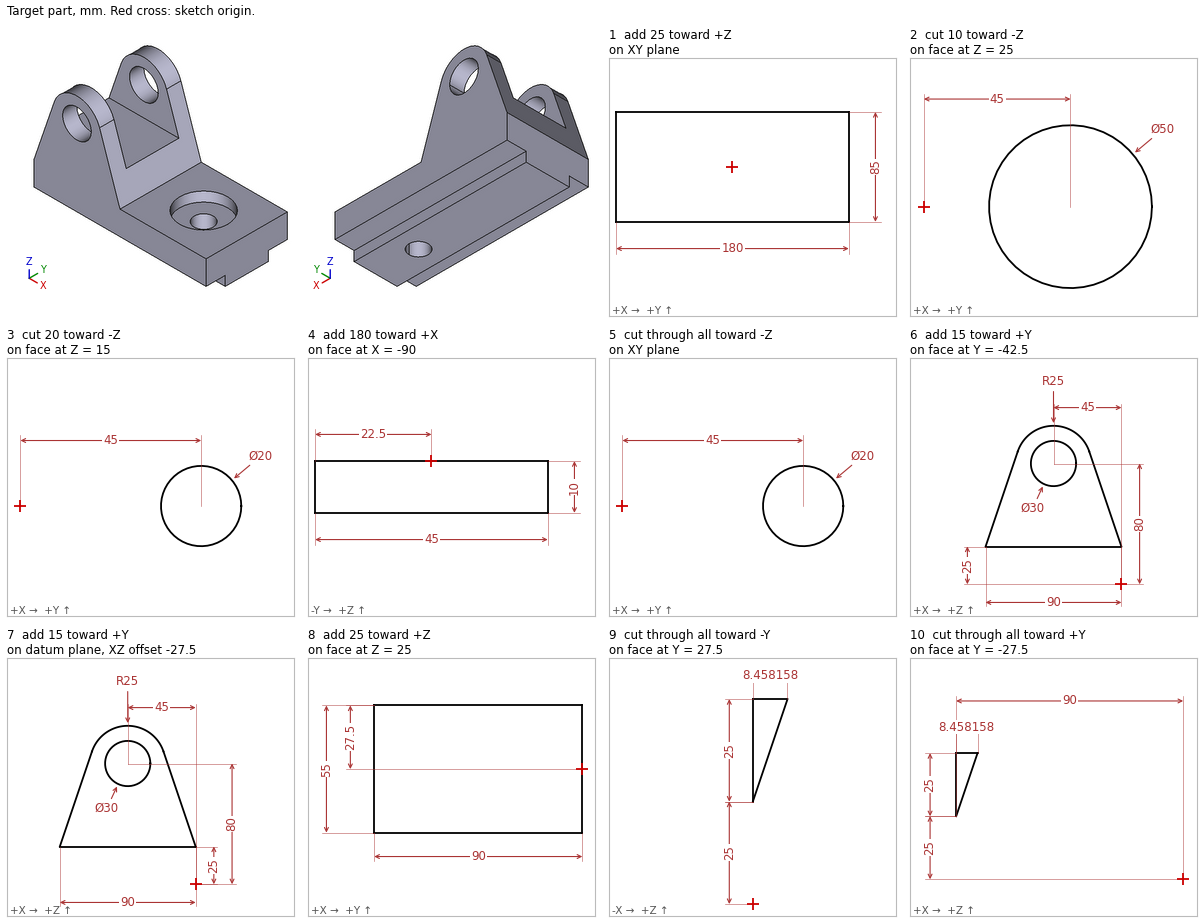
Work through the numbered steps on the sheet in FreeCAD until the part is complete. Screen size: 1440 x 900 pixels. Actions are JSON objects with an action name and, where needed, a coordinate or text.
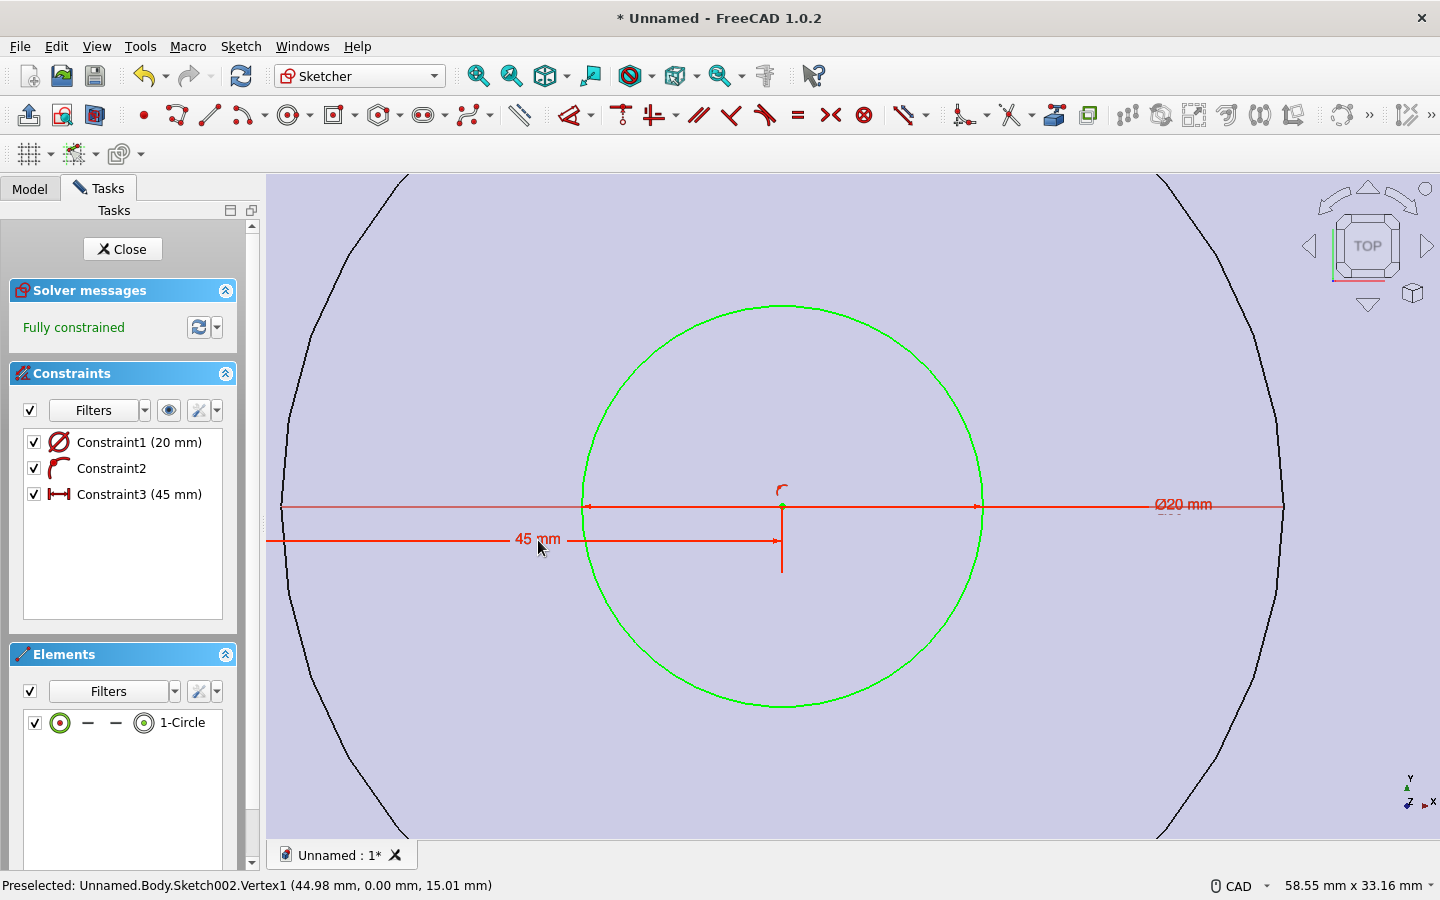
{"action": "left_click", "coordinate": [123, 249]}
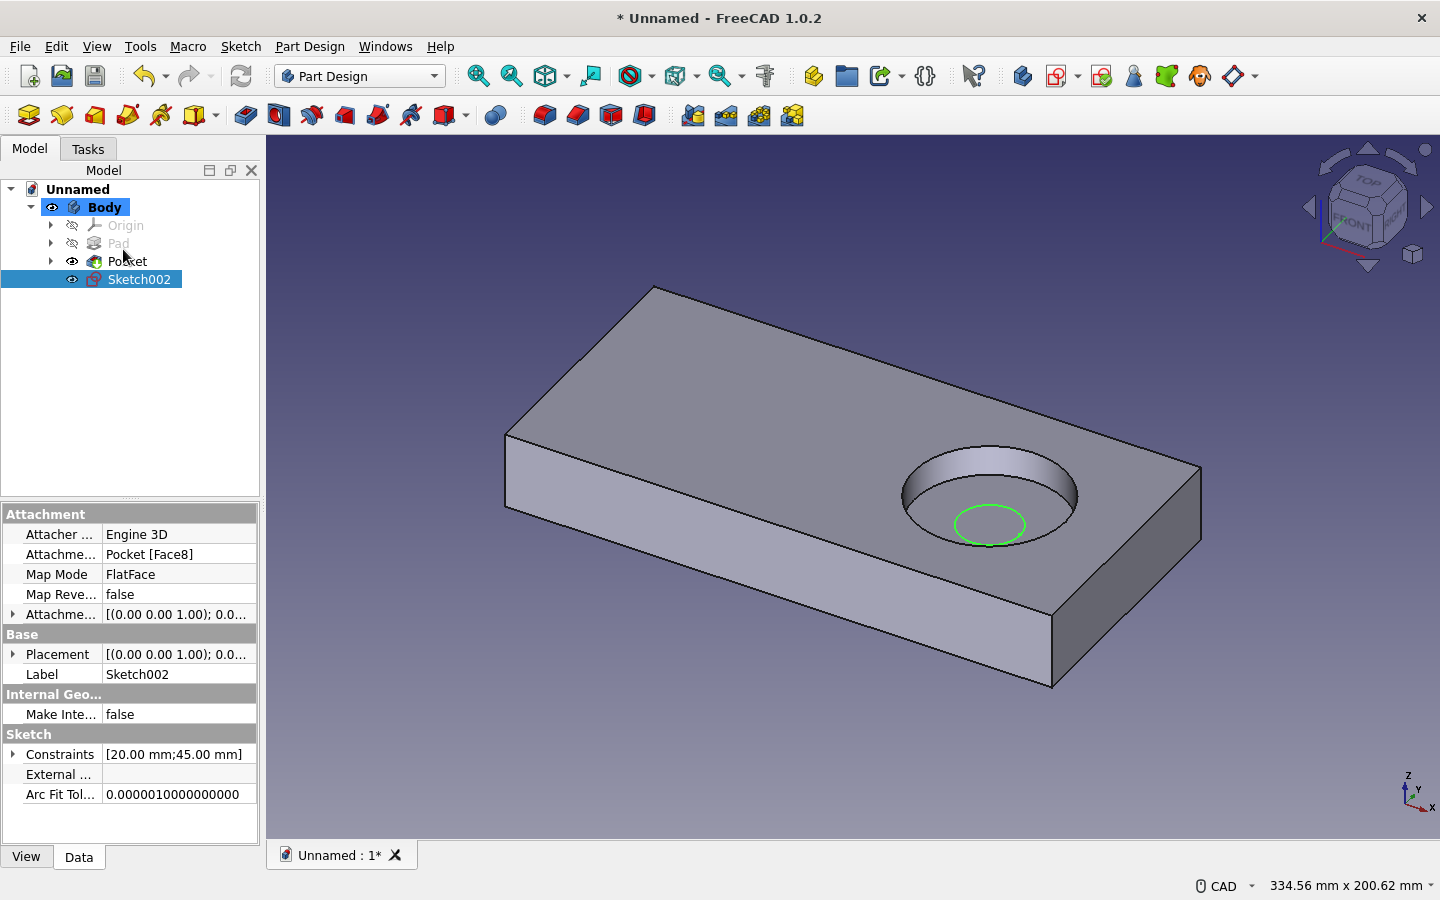
{"action": "left_click", "coordinate": [246, 116]}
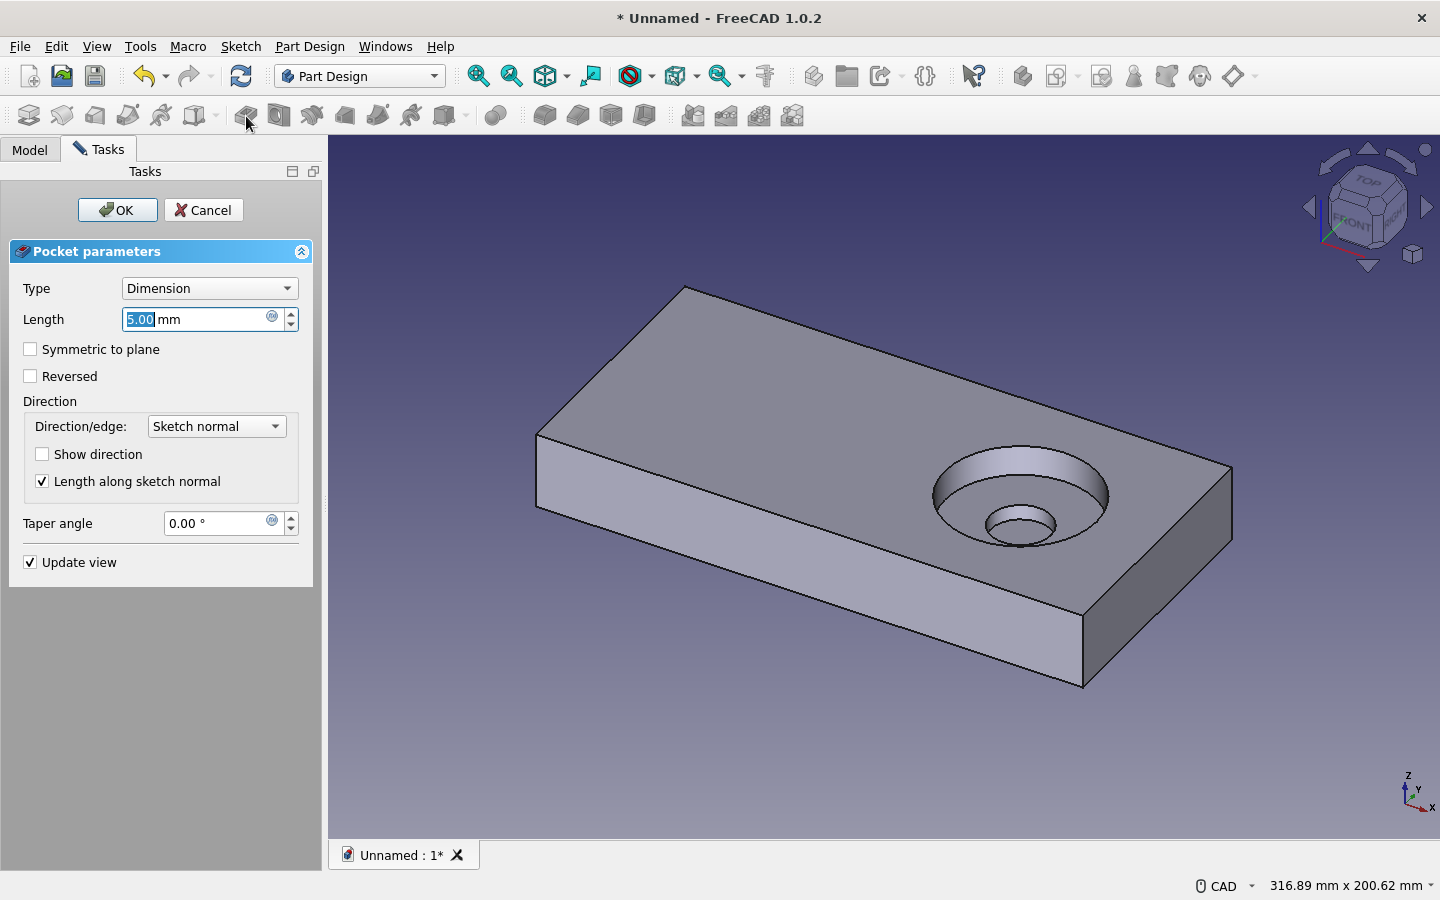
{"action": "type", "text": "20"}
{"action": "key", "text": "Tab"}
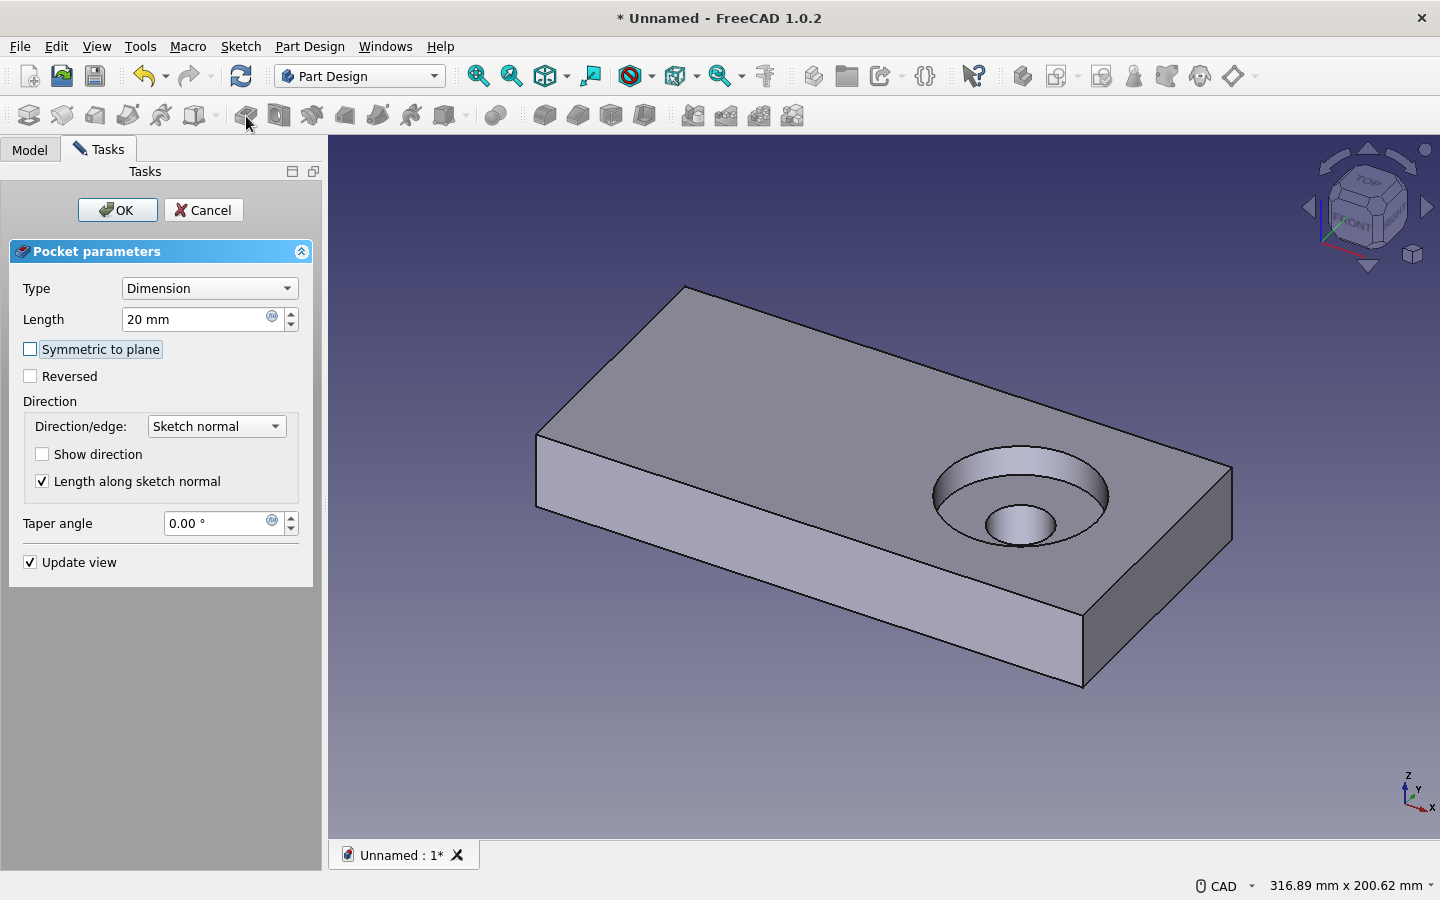
{"action": "left_click", "coordinate": [118, 210]}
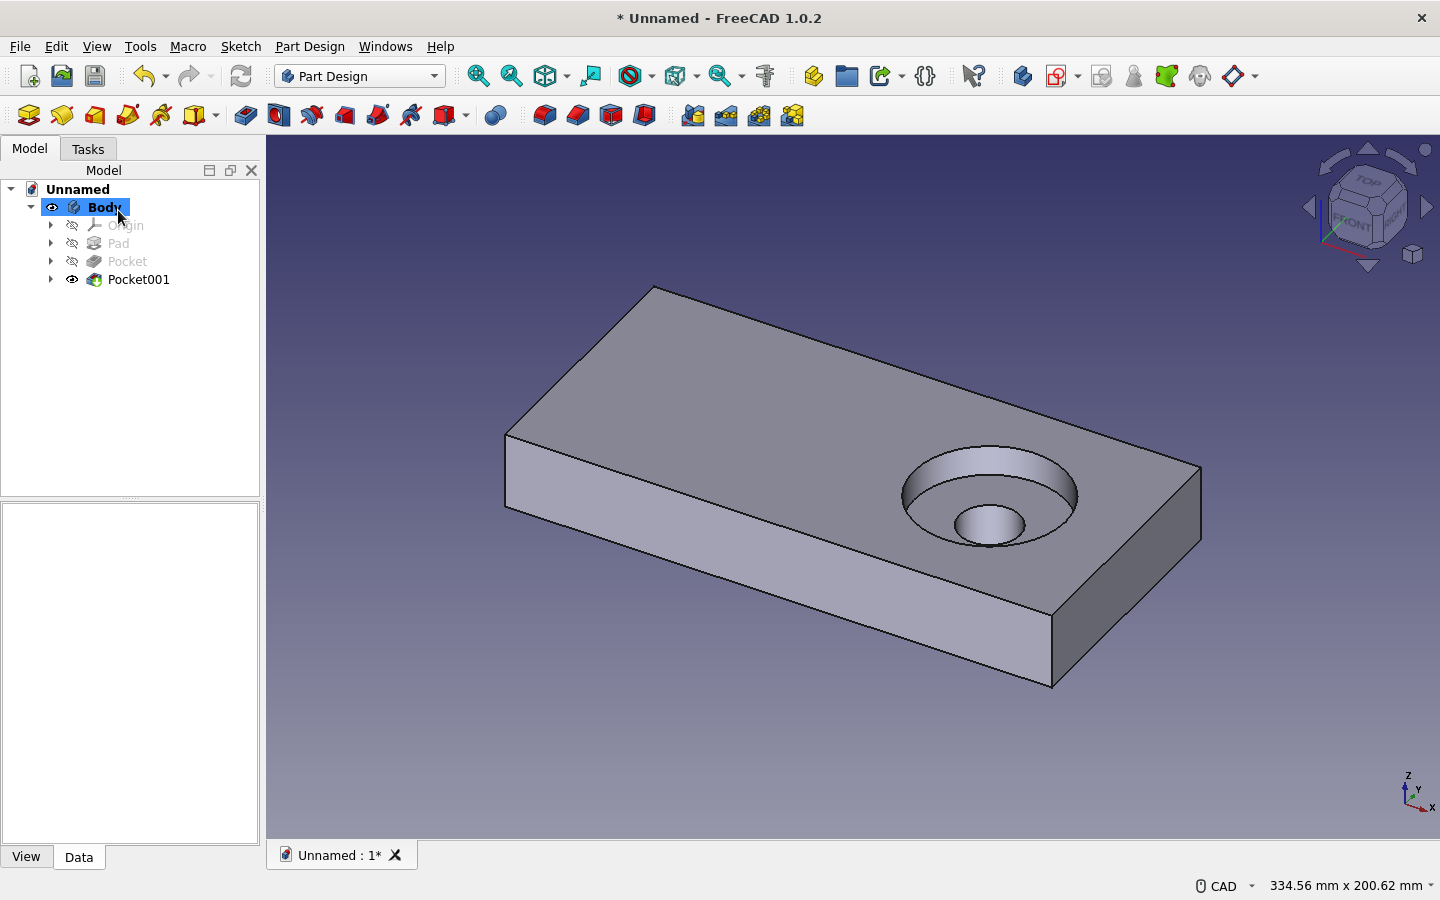
{"action": "key", "text": "6"}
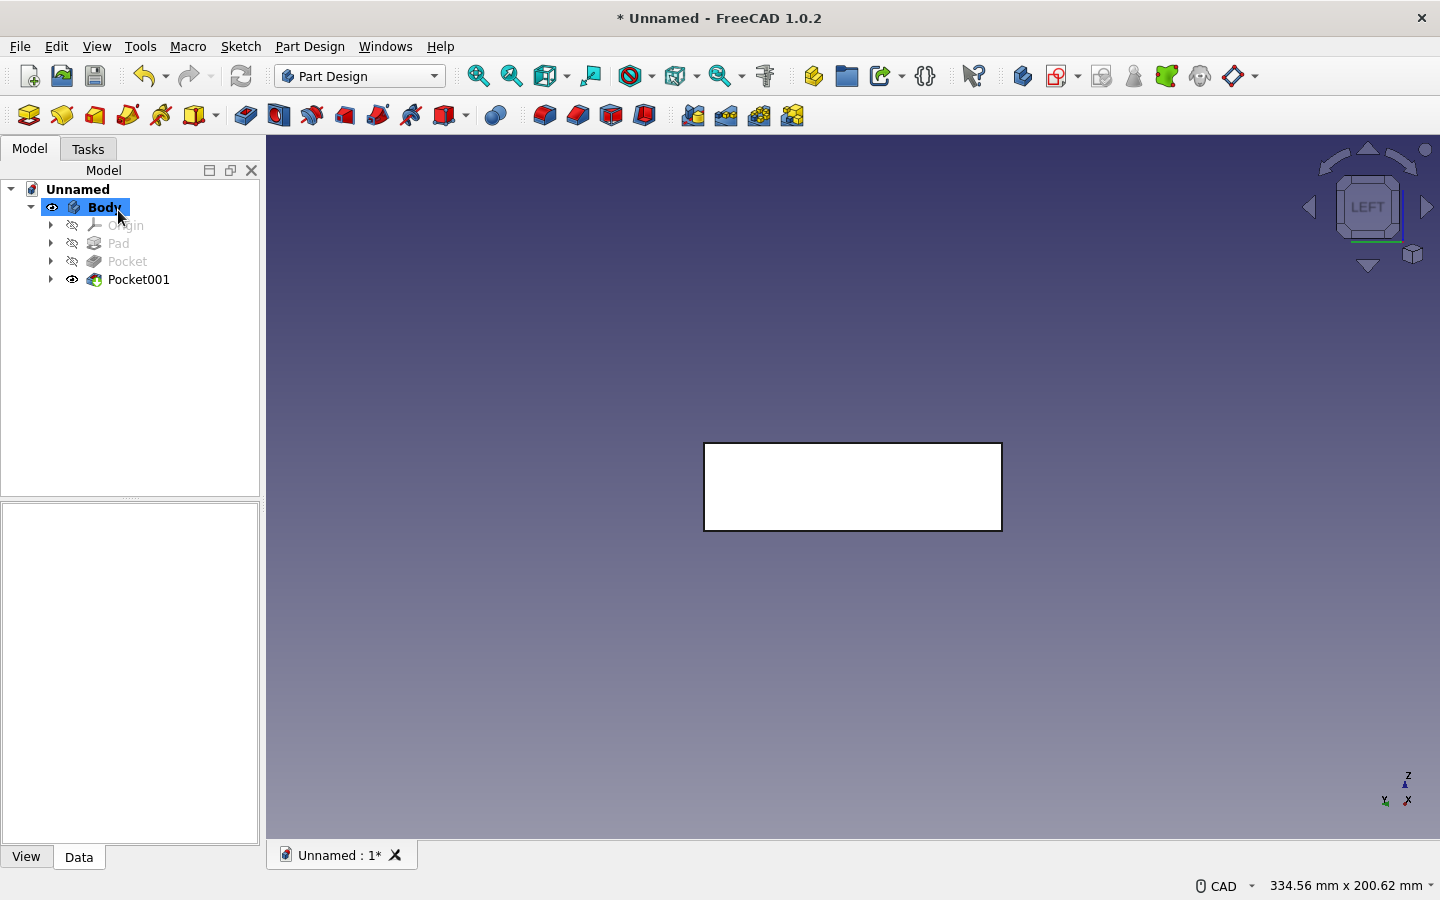
{"action": "left_click", "coordinate": [479, 76]}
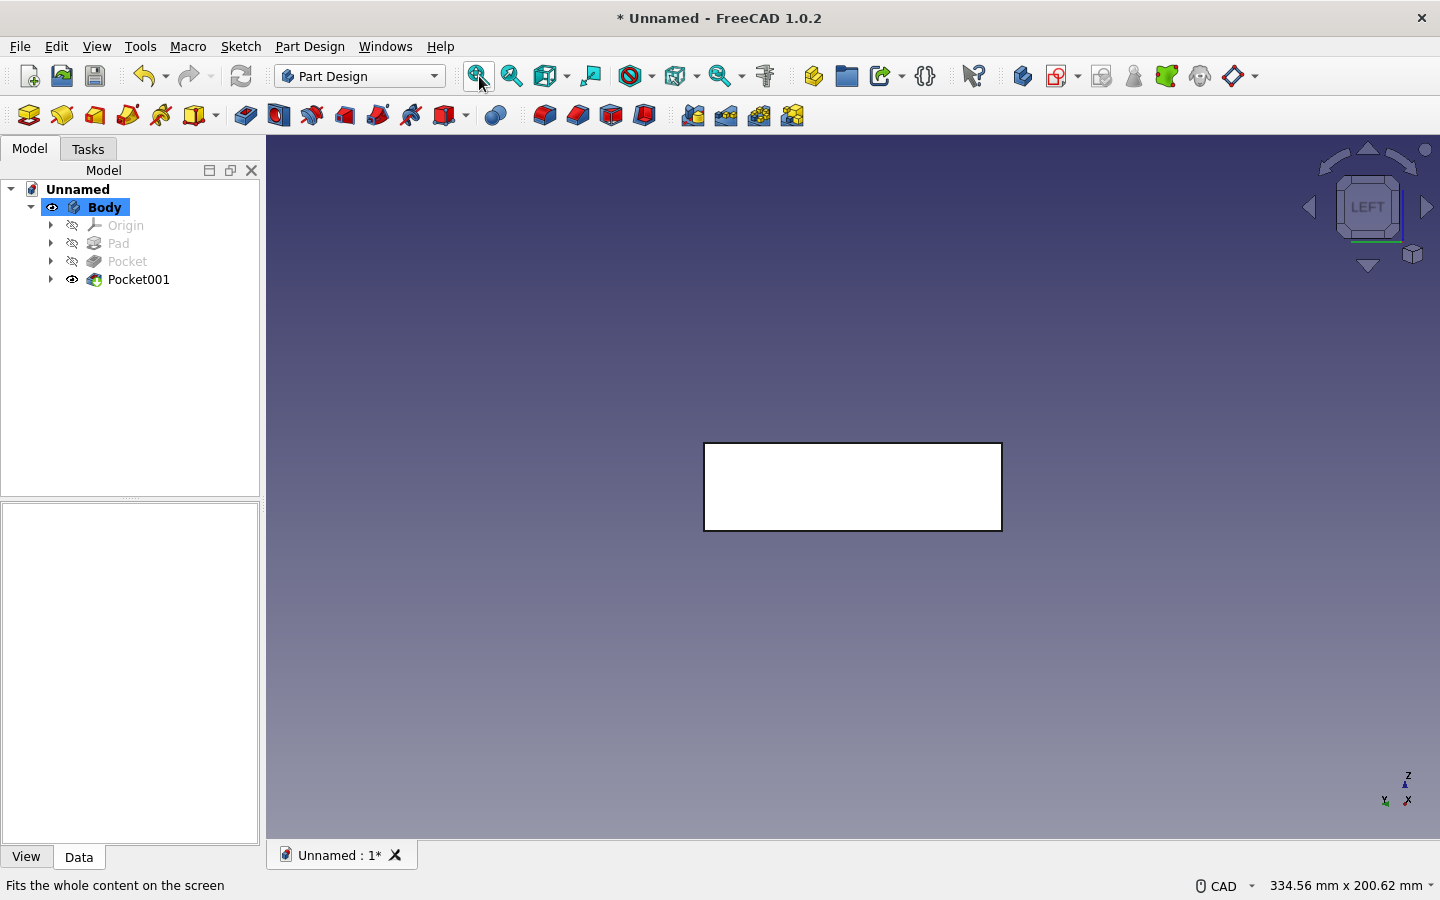
{"action": "left_click", "coordinate": [768, 486]}